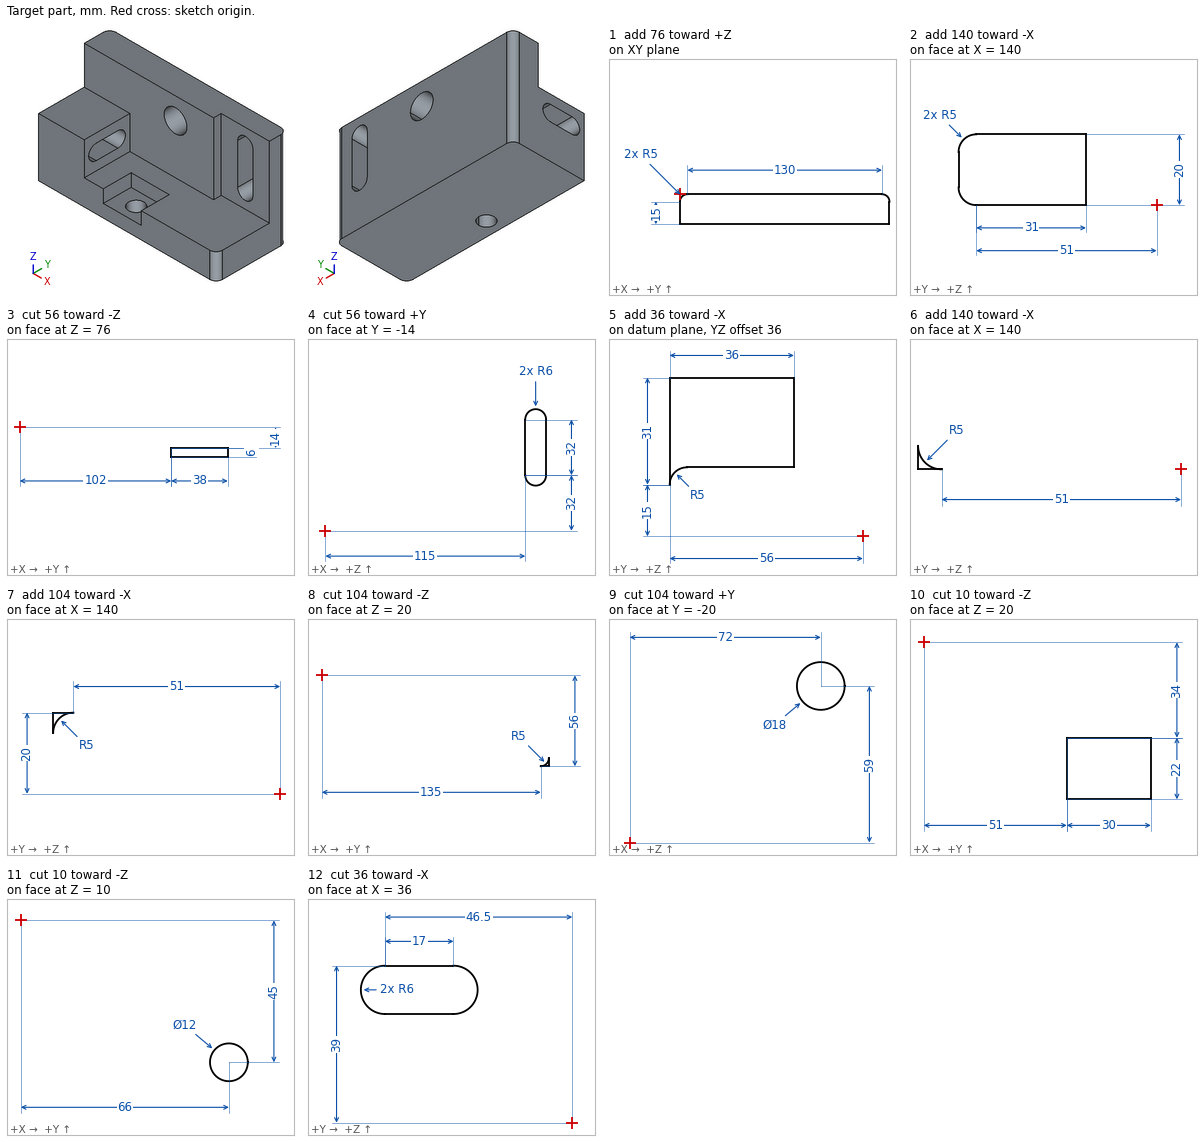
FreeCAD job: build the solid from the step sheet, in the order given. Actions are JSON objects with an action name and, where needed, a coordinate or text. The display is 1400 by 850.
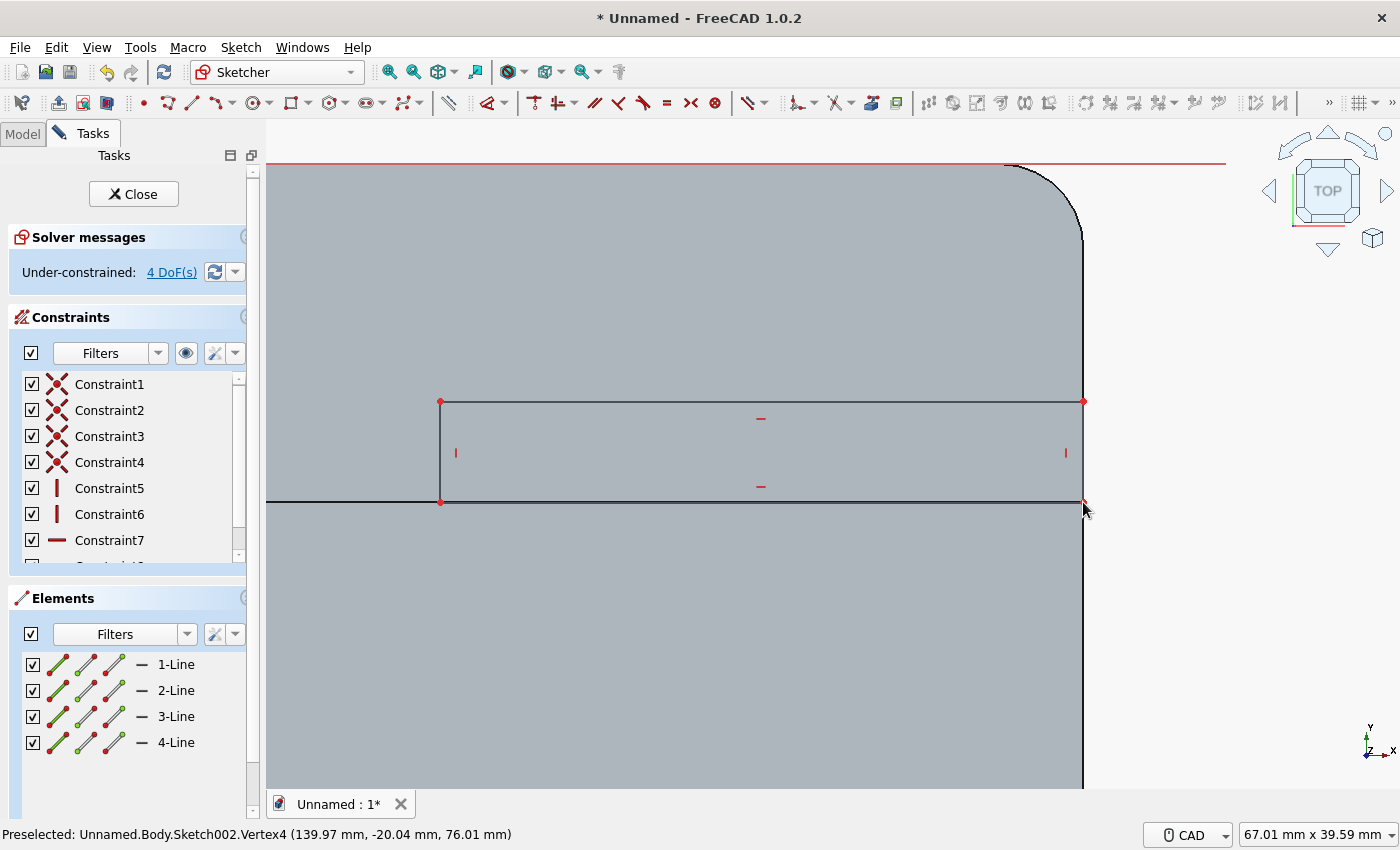
{"action": "left_click", "coordinate": [488, 104]}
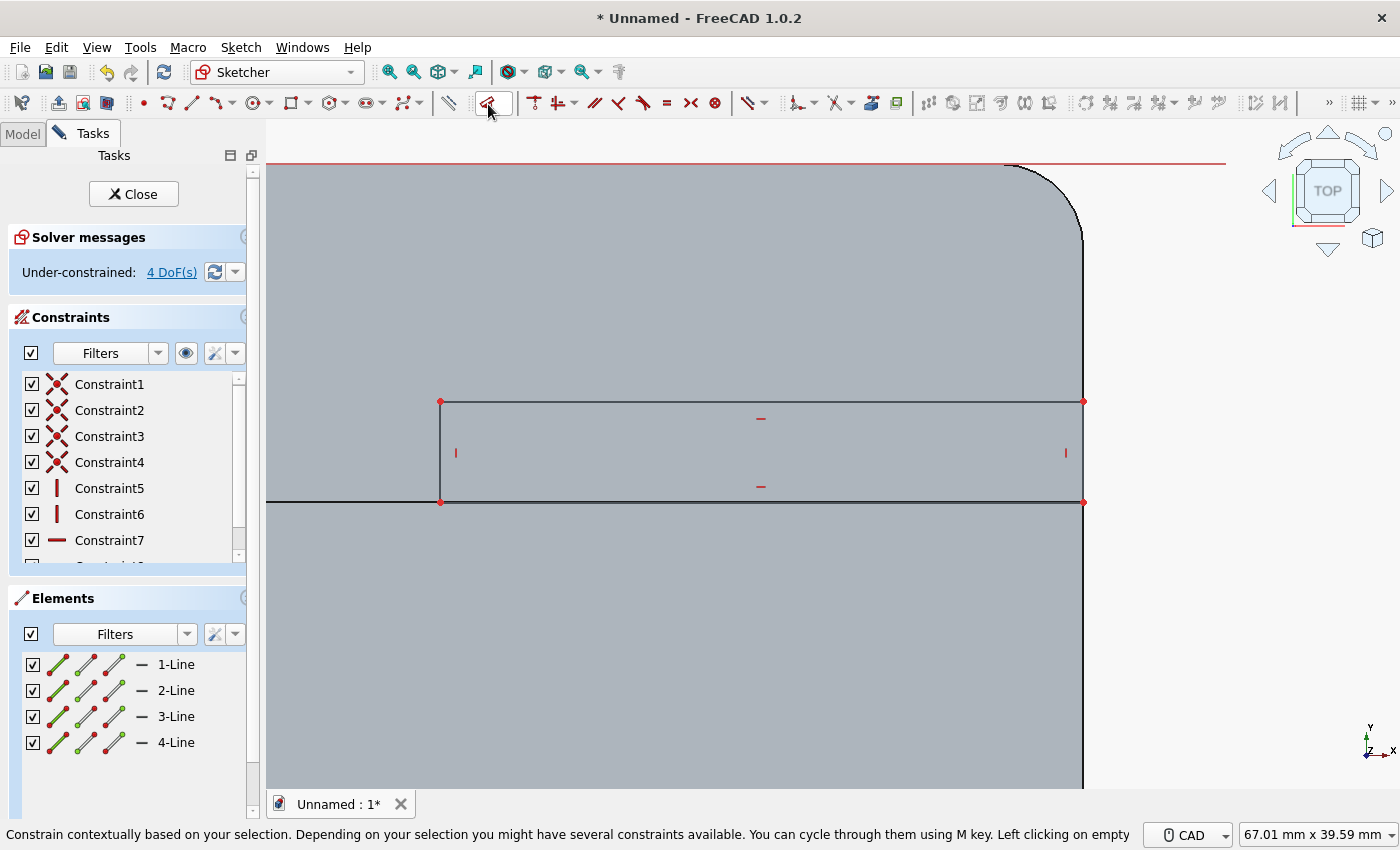
{"action": "left_click", "coordinate": [440, 432]}
{"action": "left_click", "coordinate": [406, 452]}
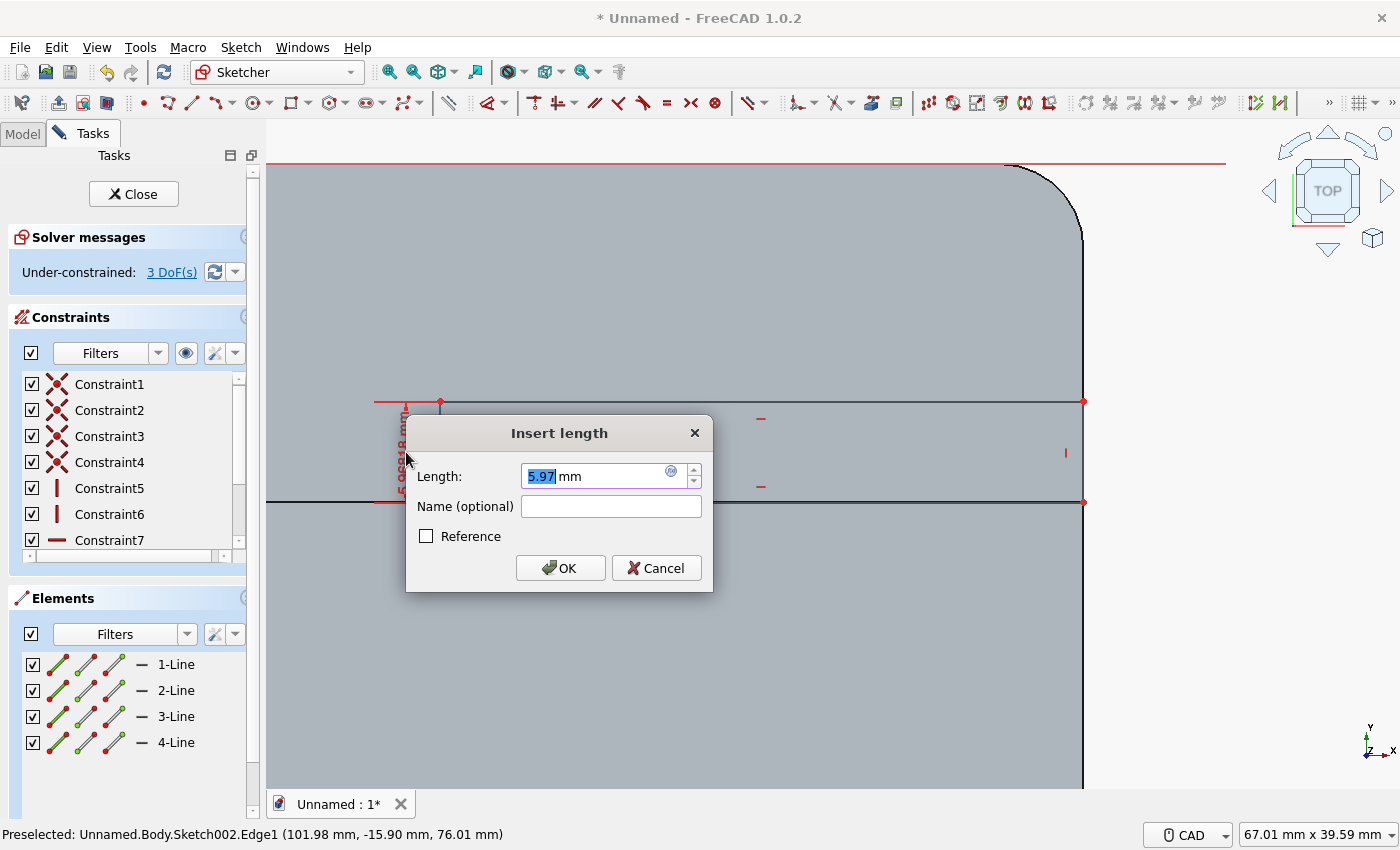
{"action": "type", "text": "6"}
{"action": "key", "text": "Return"}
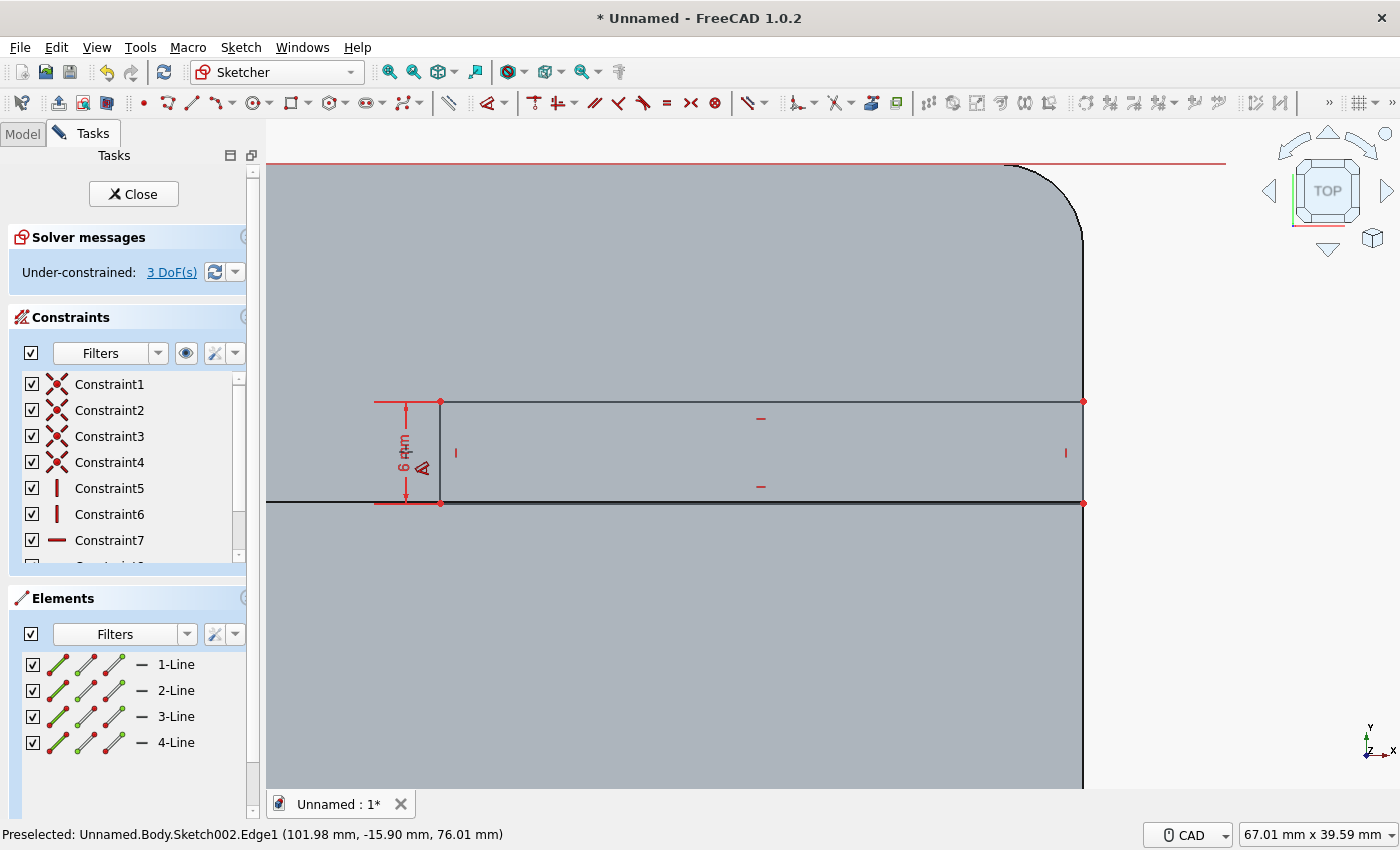
{"action": "left_click", "coordinate": [633, 504]}
{"action": "left_click", "coordinate": [762, 538]}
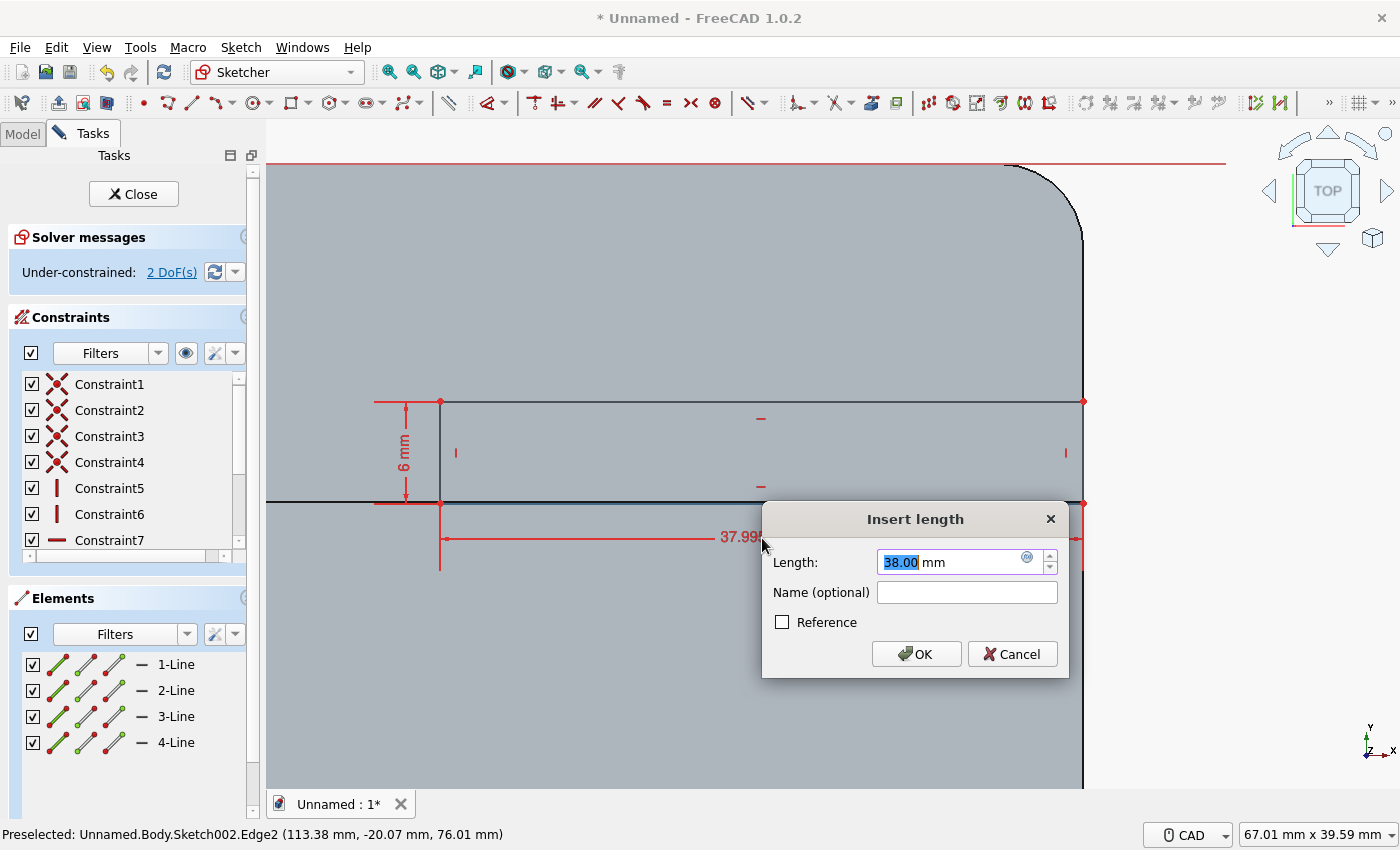
{"action": "type", "text": "38"}
{"action": "key", "text": "Return"}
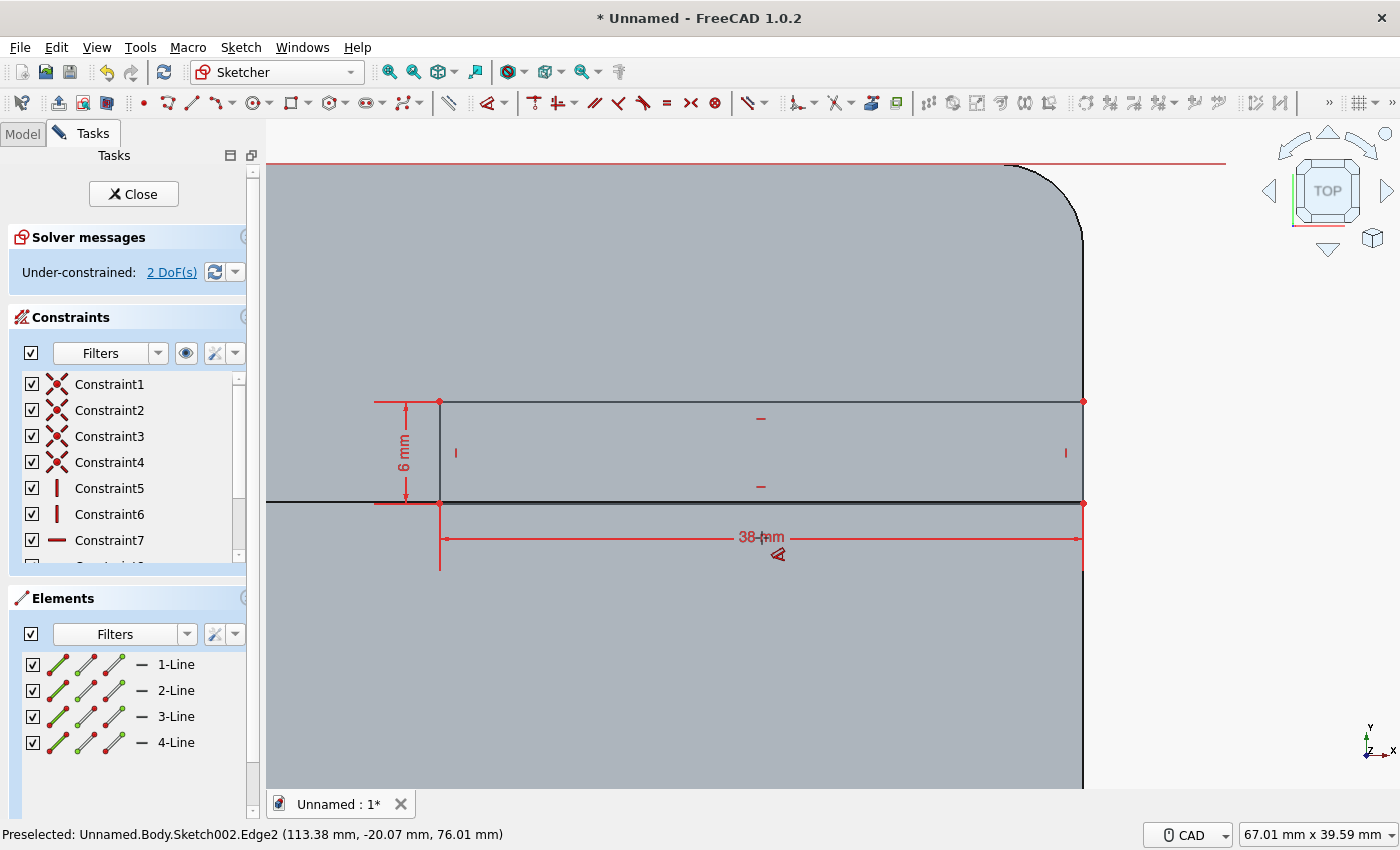
{"action": "left_click", "coordinate": [440, 402]}
{"action": "left_click", "coordinate": [474, 283]}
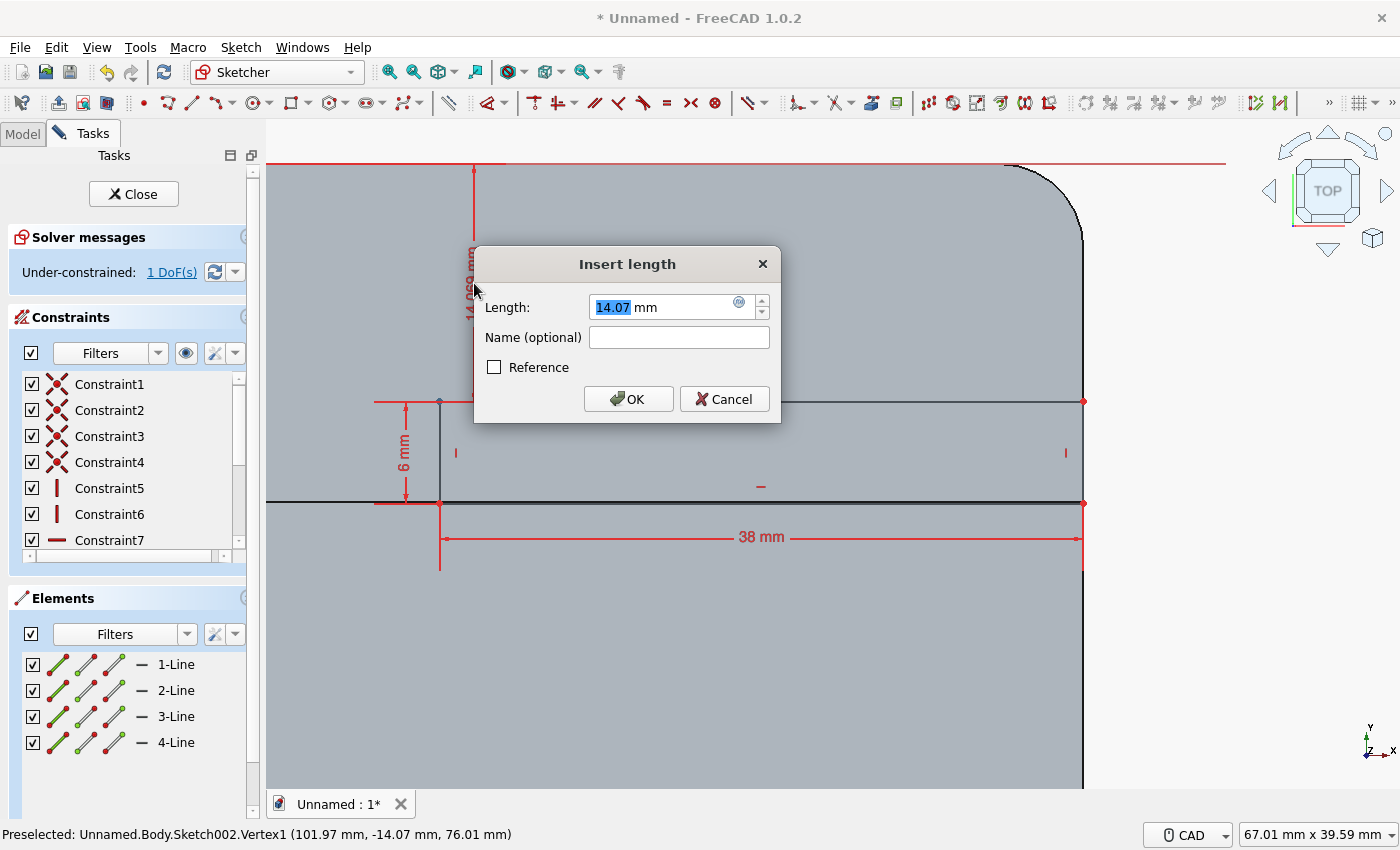
{"action": "type", "text": "14"}
{"action": "key", "text": "Return"}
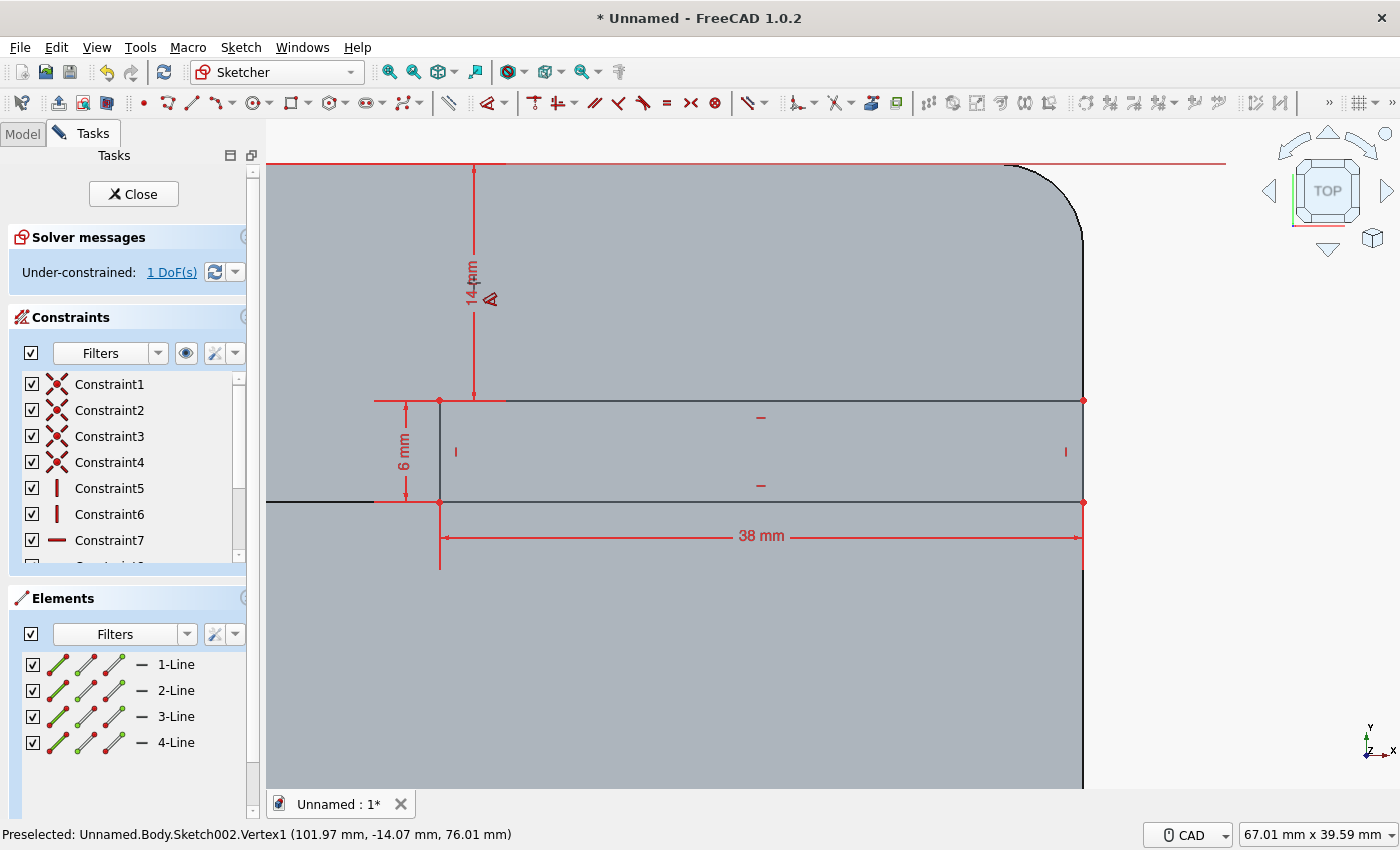
{"action": "left_click", "coordinate": [440, 401]}
{"action": "left_click", "coordinate": [333, 435]}